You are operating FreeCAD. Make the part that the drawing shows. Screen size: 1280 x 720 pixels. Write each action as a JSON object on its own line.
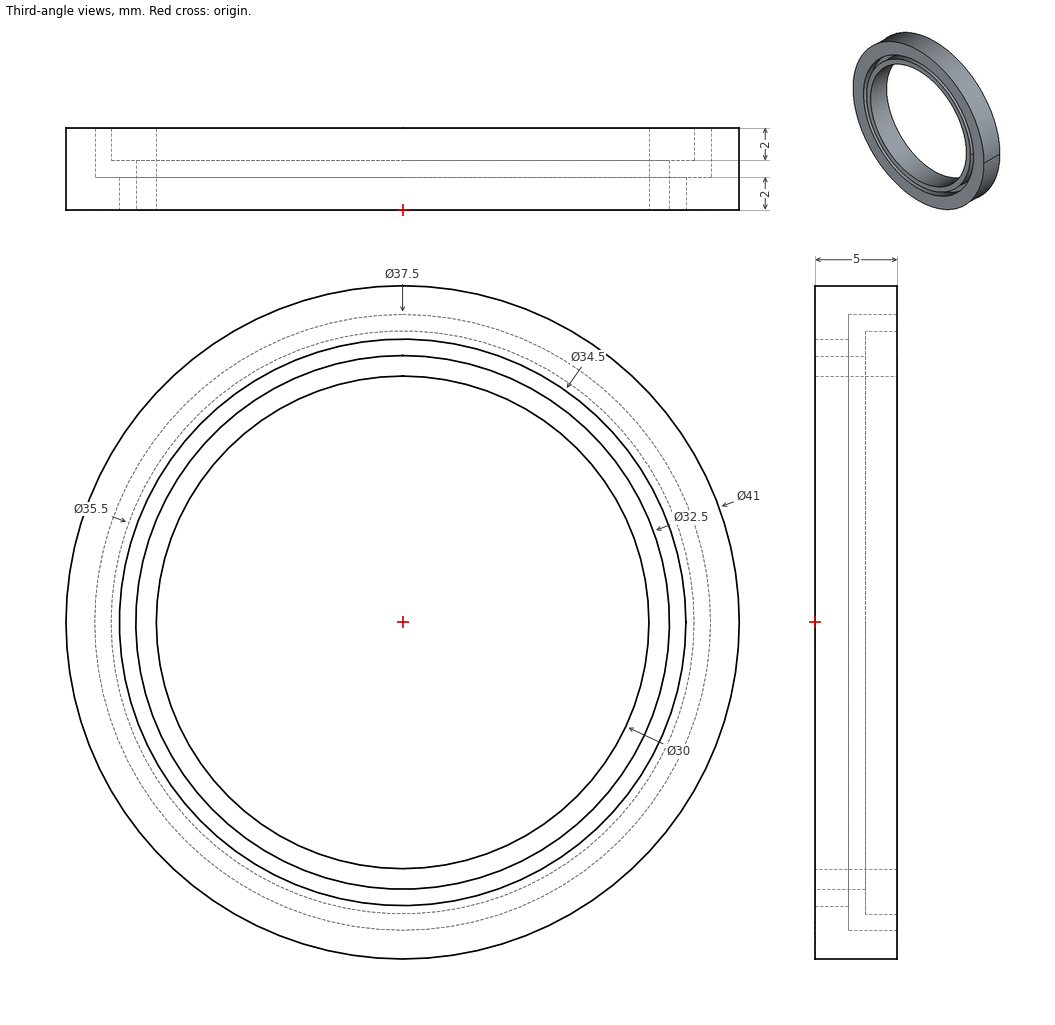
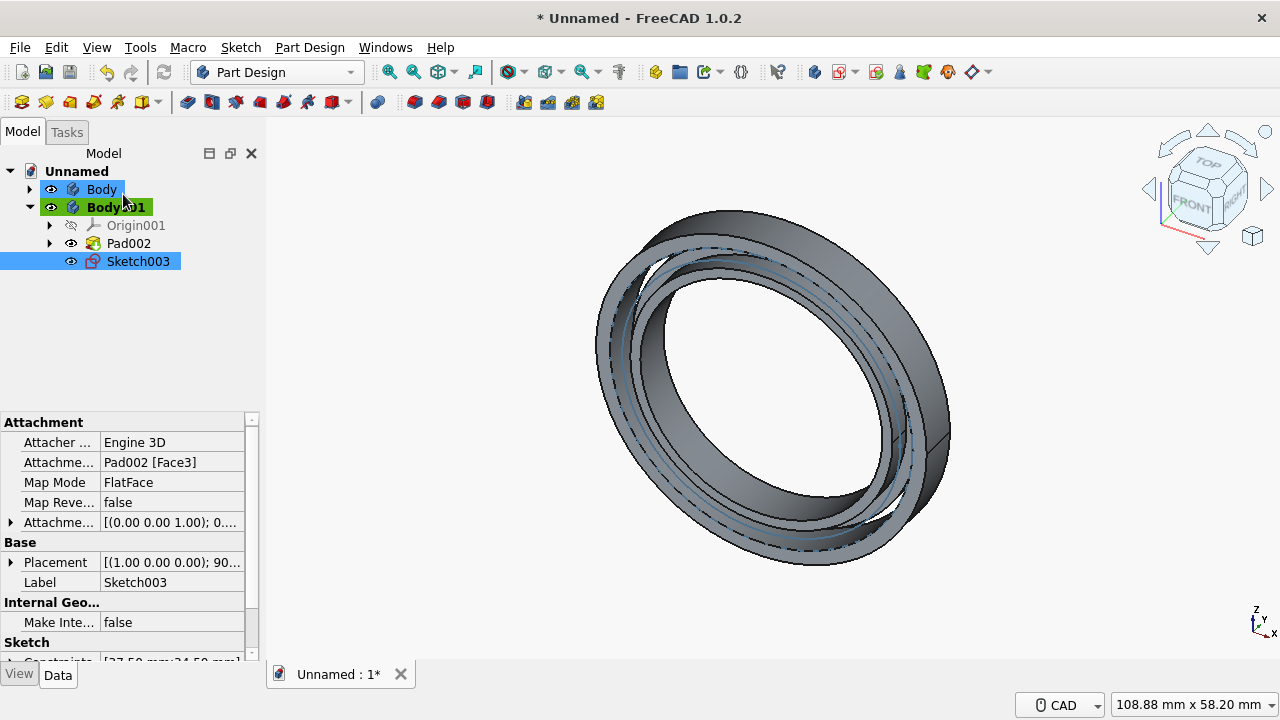
{"action": "left_click", "coordinate": [22, 102]}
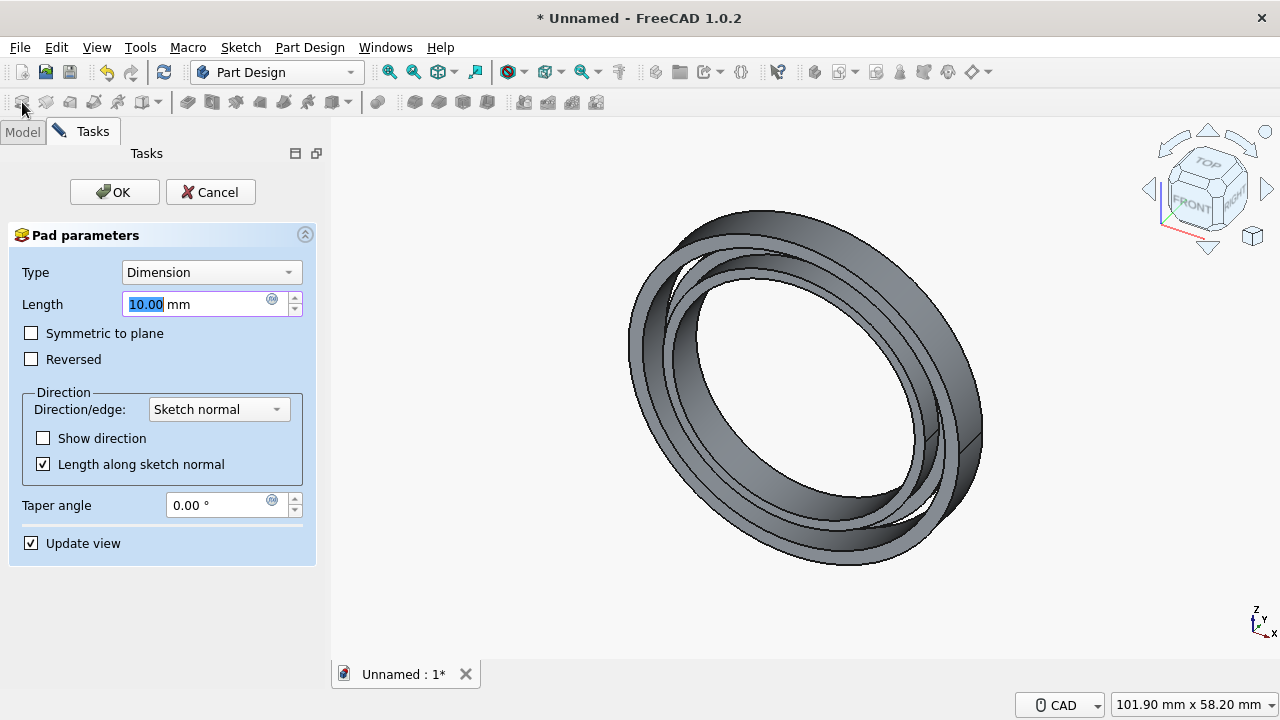
{"action": "type", "text": "2"}
{"action": "key", "text": "Tab"}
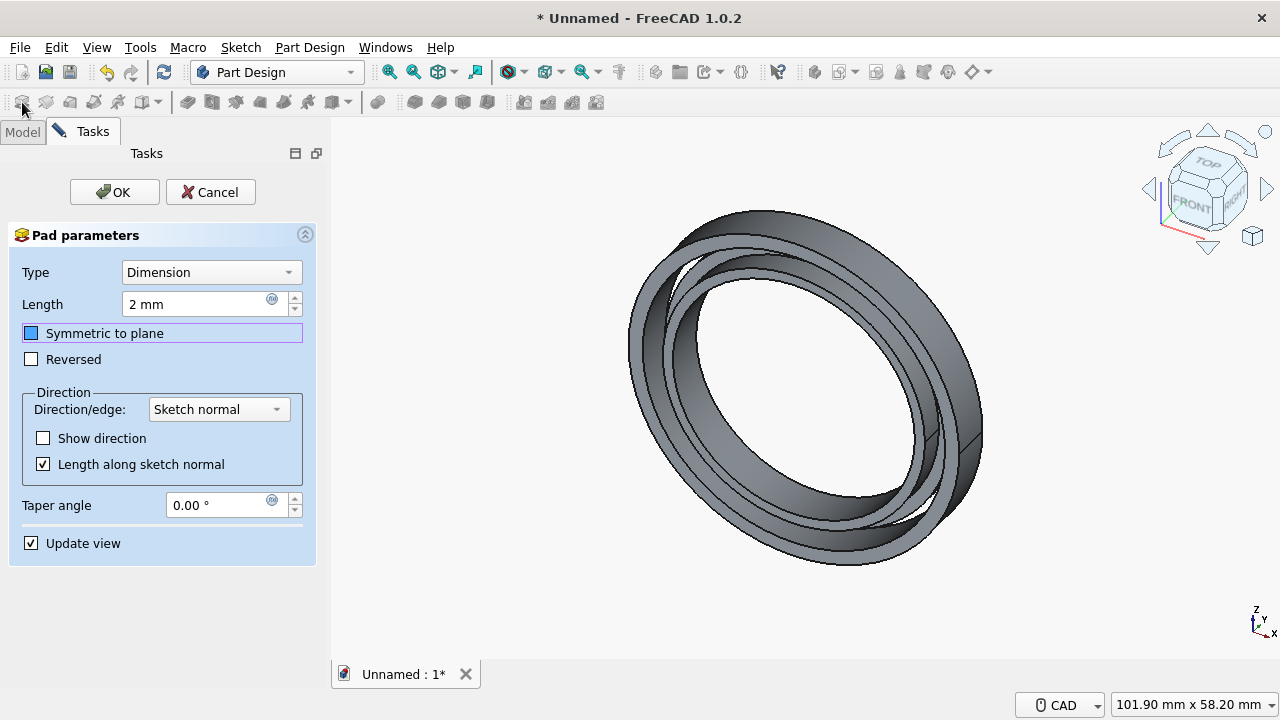
{"action": "left_click", "coordinate": [30, 359]}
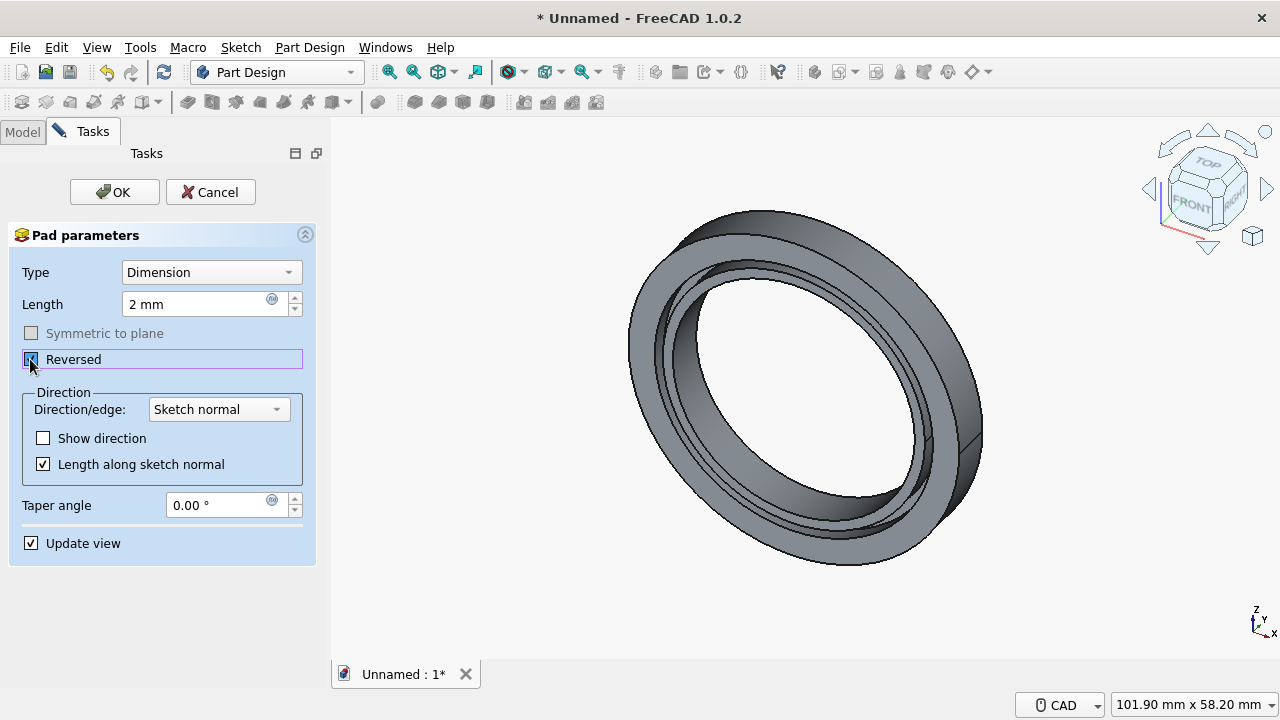
{"action": "left_click", "coordinate": [115, 192]}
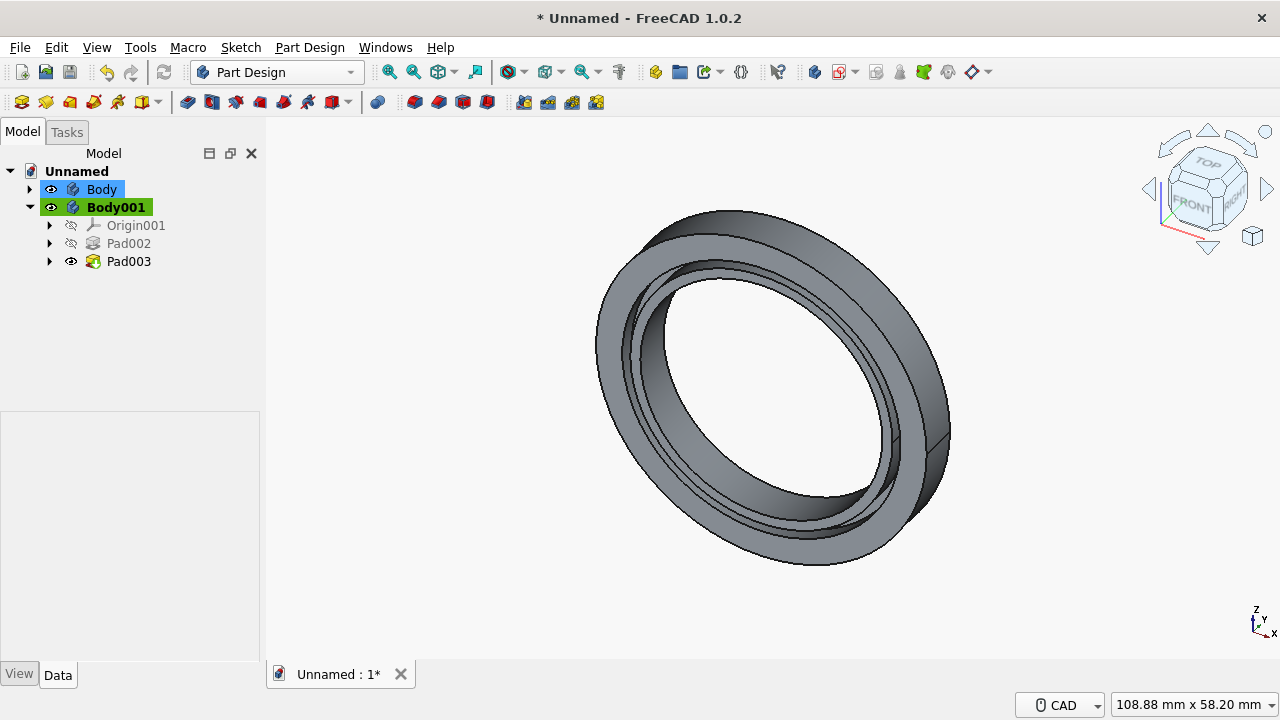
{"action": "key", "text": "0"}